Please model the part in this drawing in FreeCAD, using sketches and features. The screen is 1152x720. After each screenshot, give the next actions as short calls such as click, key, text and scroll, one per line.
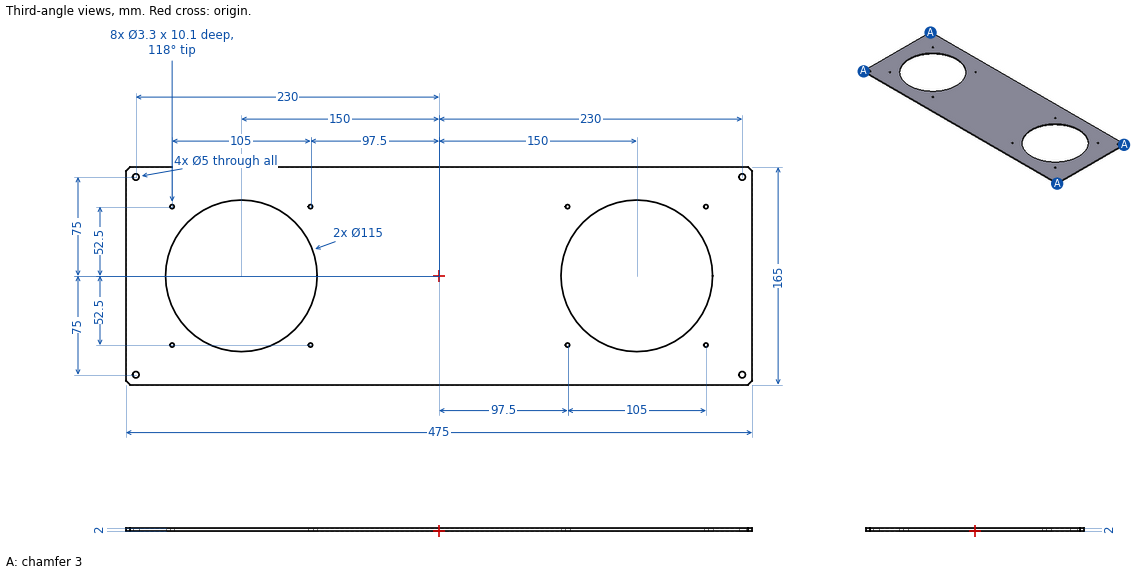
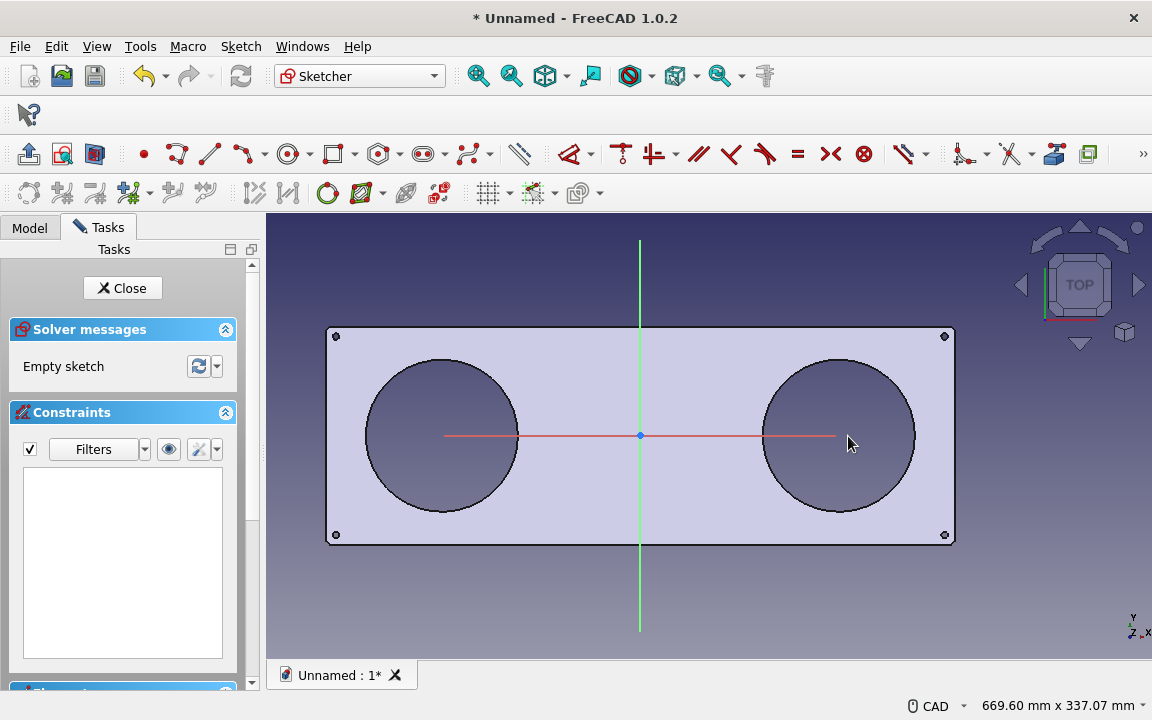
click(288, 154)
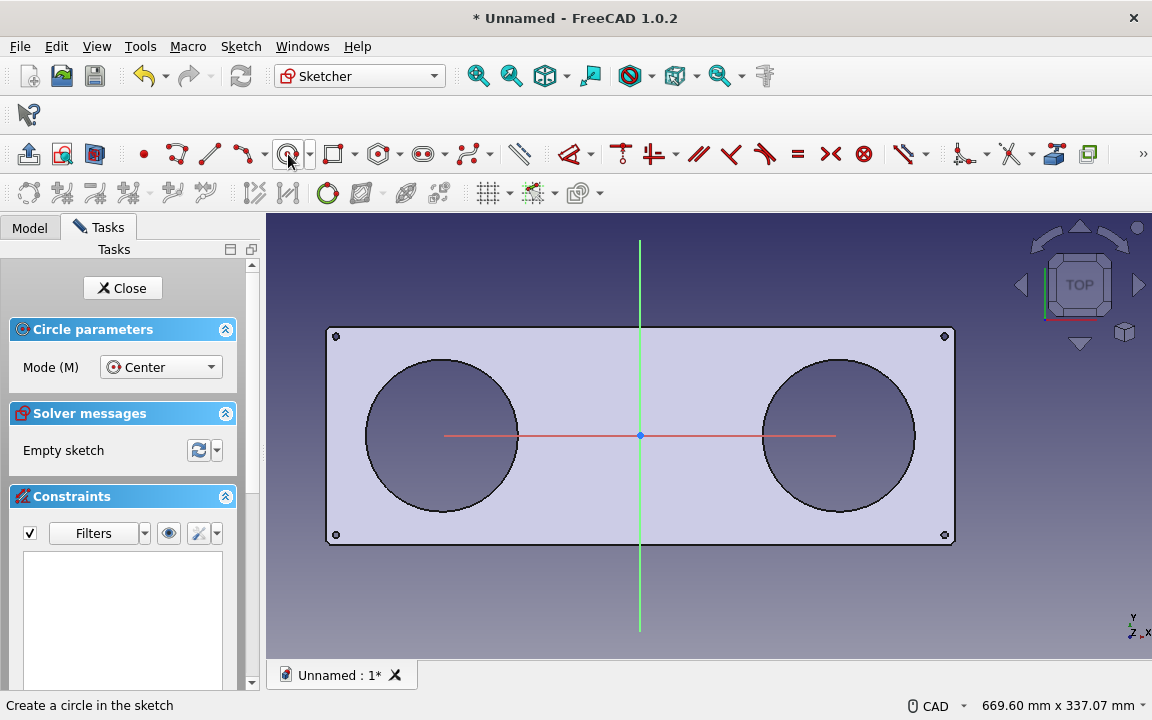
scroll(372, 366, up, 12)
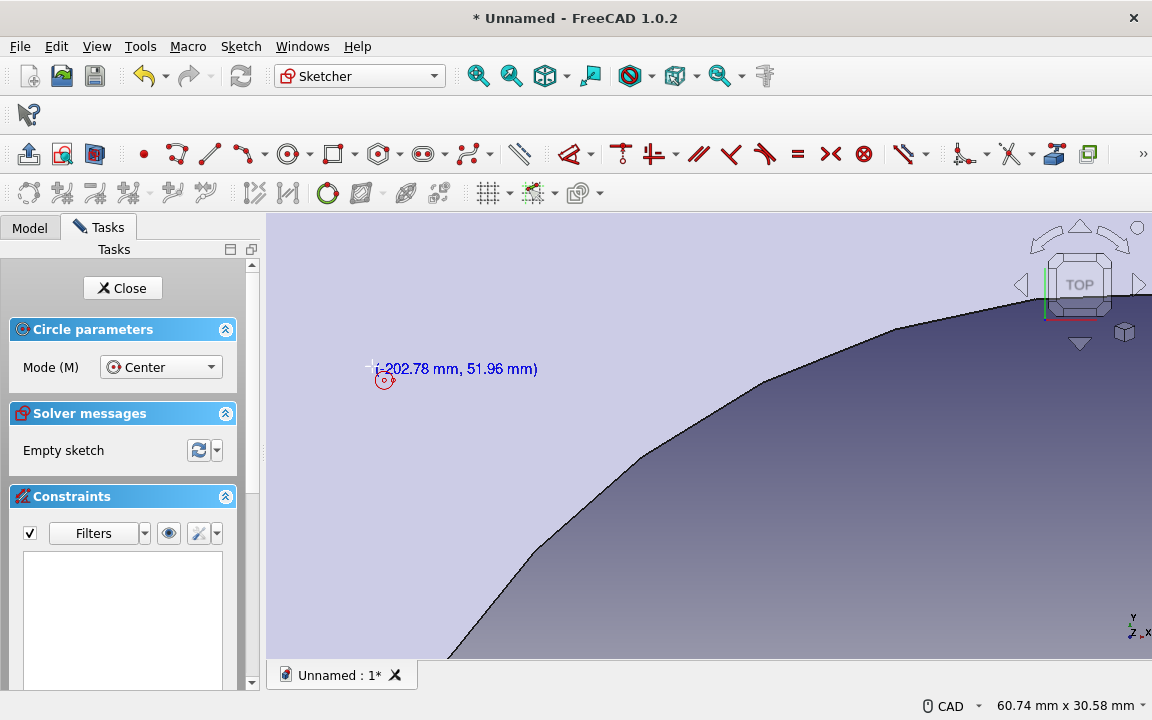
scroll(372, 367, down, 12)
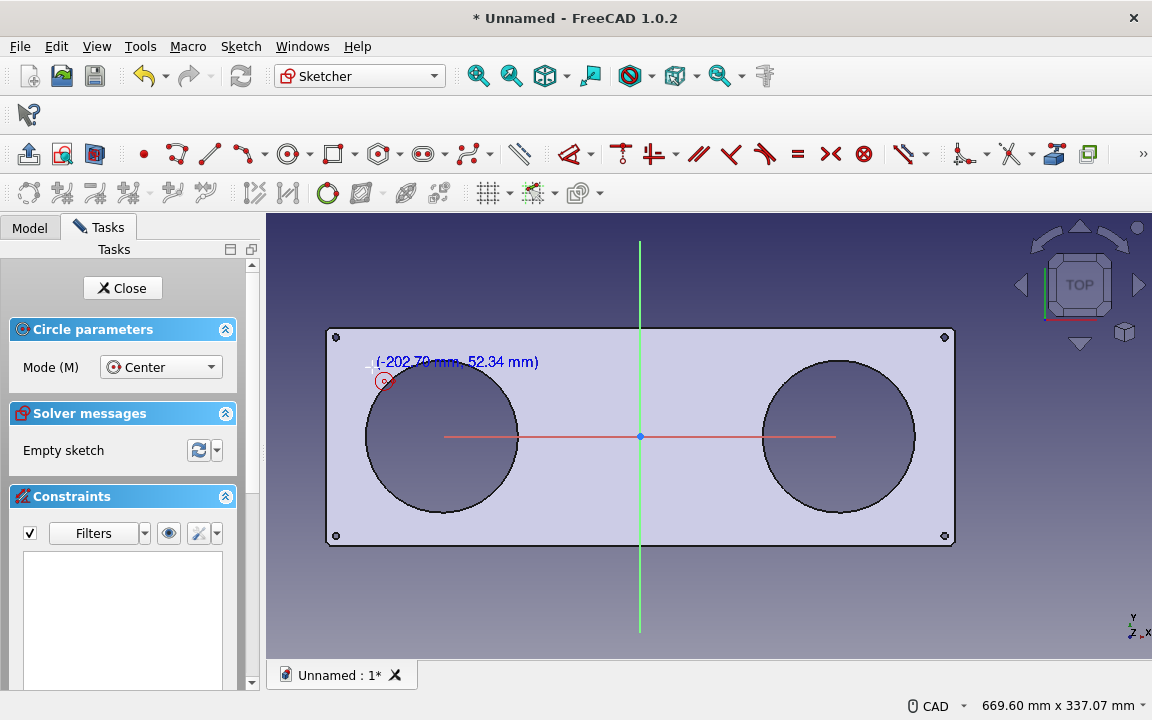
click(372, 367)
move(374, 366)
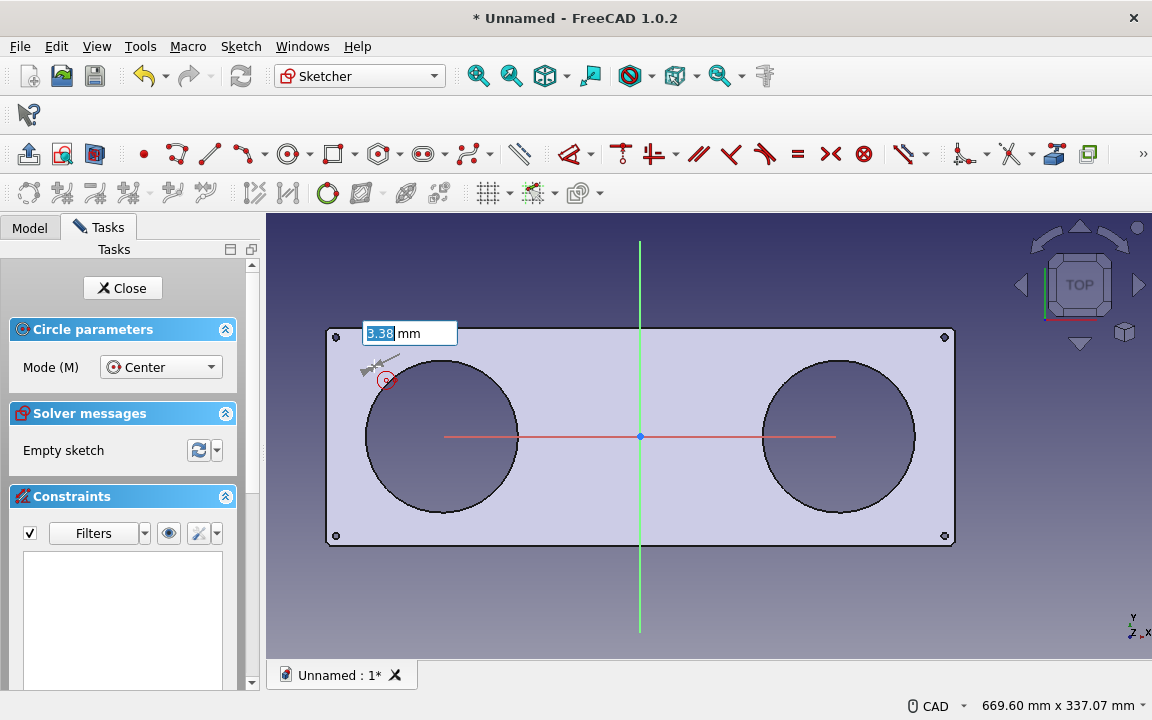
text(3.3)
key(Return)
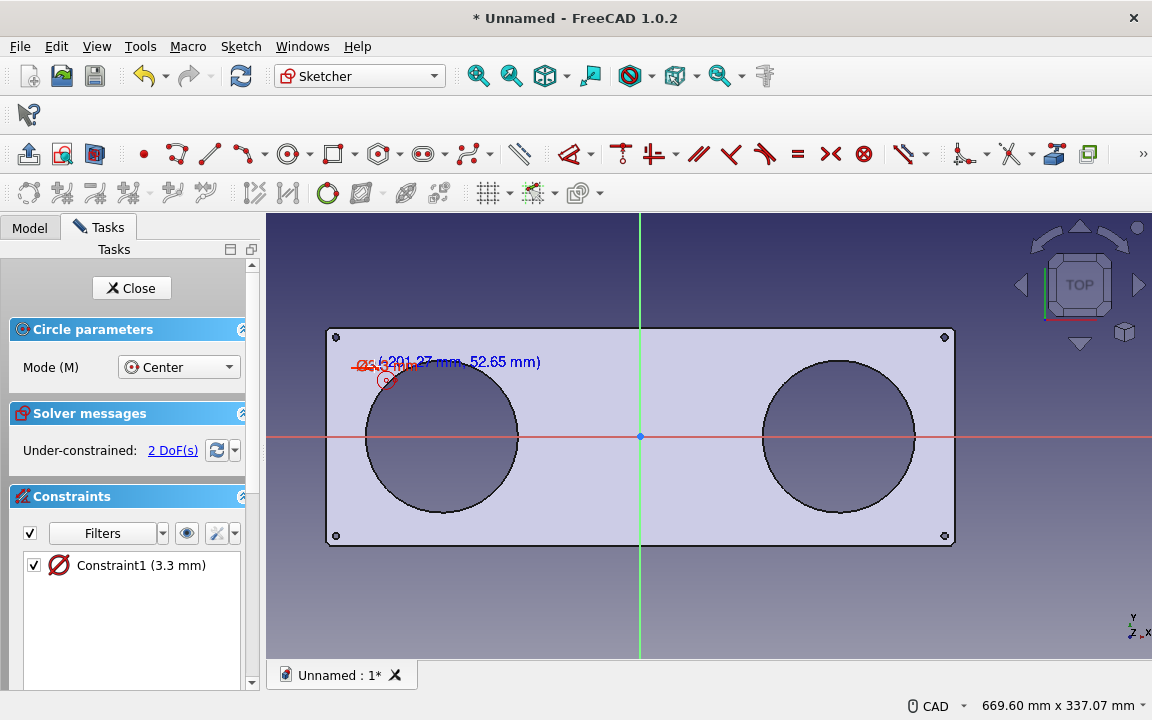
scroll(511, 367, up, 12)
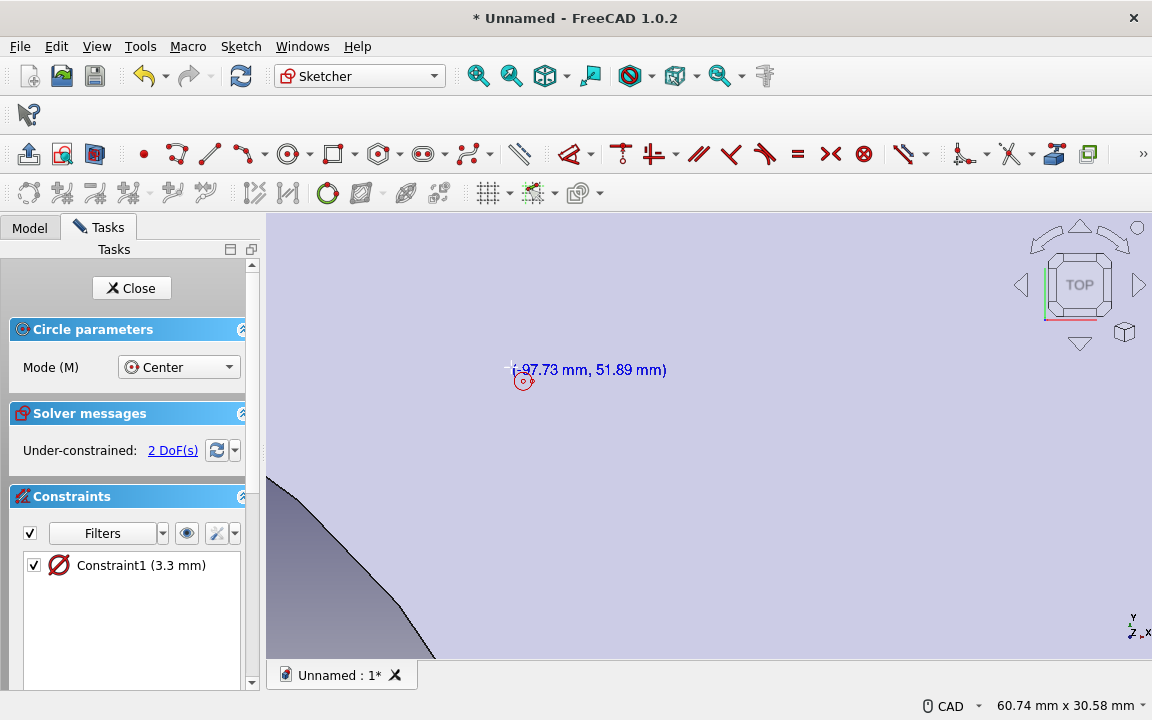
scroll(511, 367, down, 12)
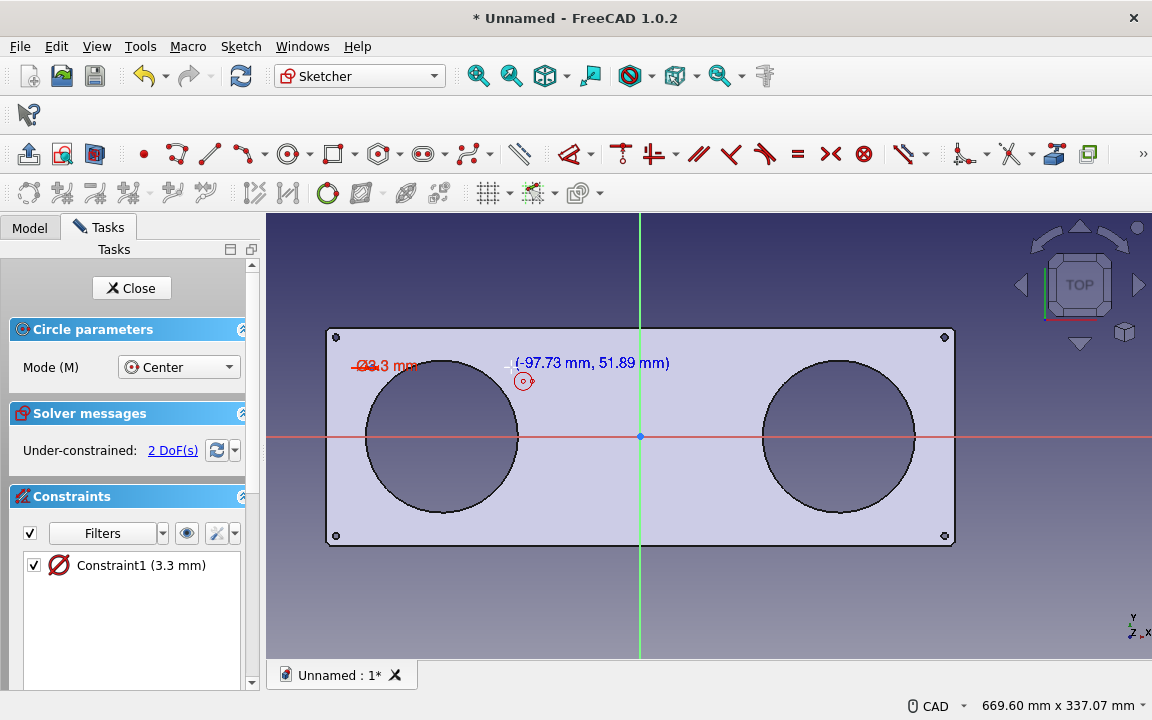
click(511, 367)
move(513, 366)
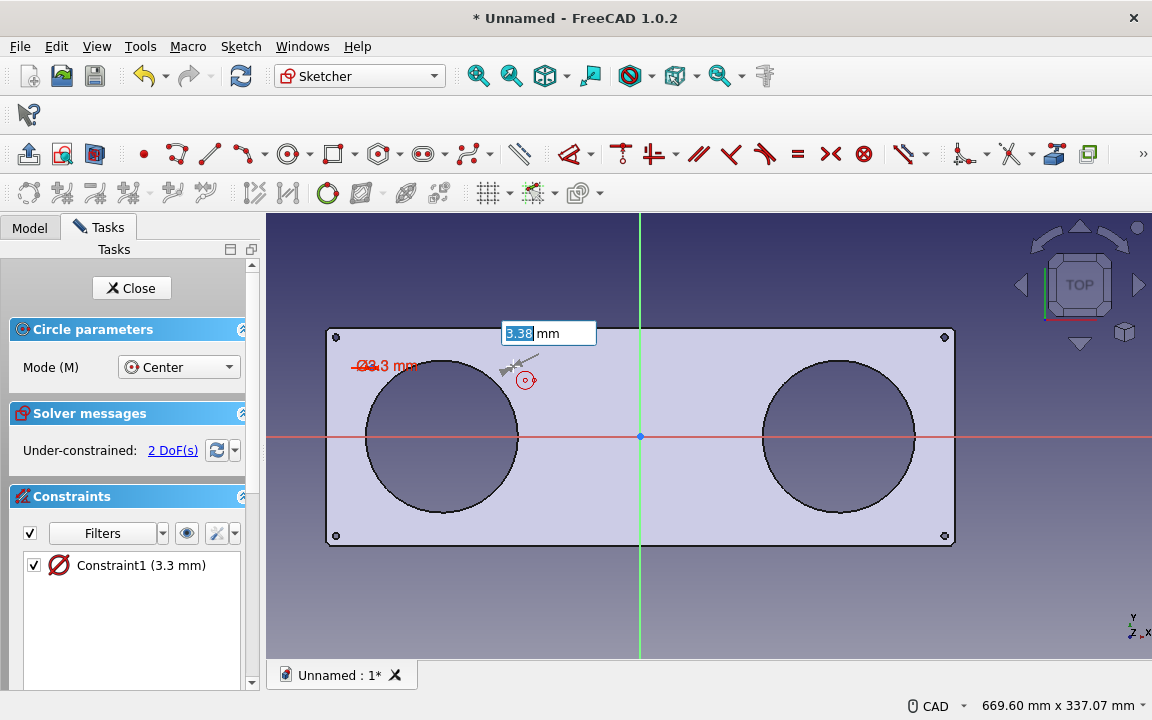
text(3.3)
key(Return)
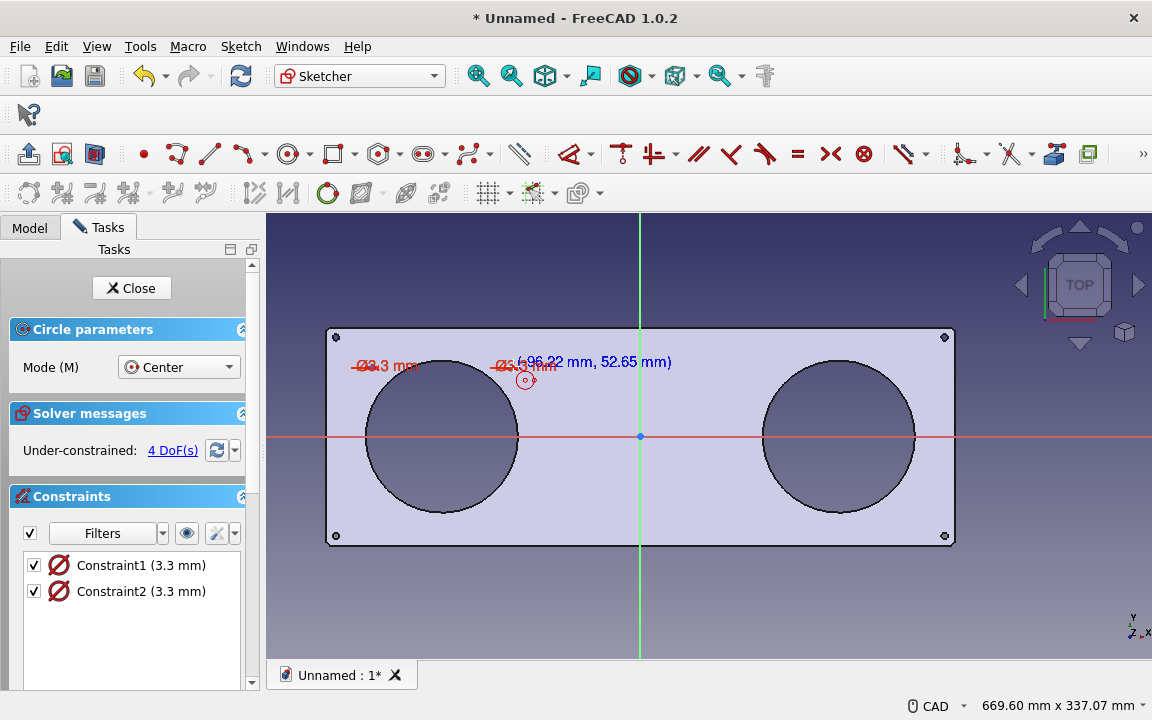
scroll(511, 506, up, 12)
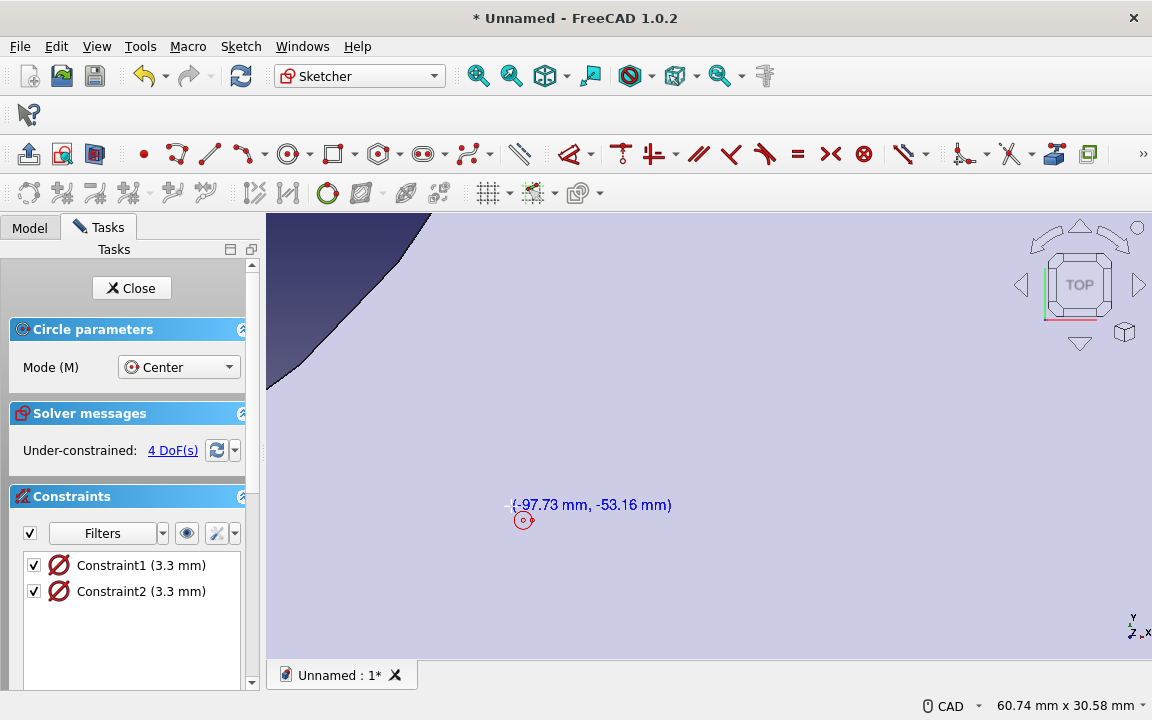
scroll(511, 506, down, 12)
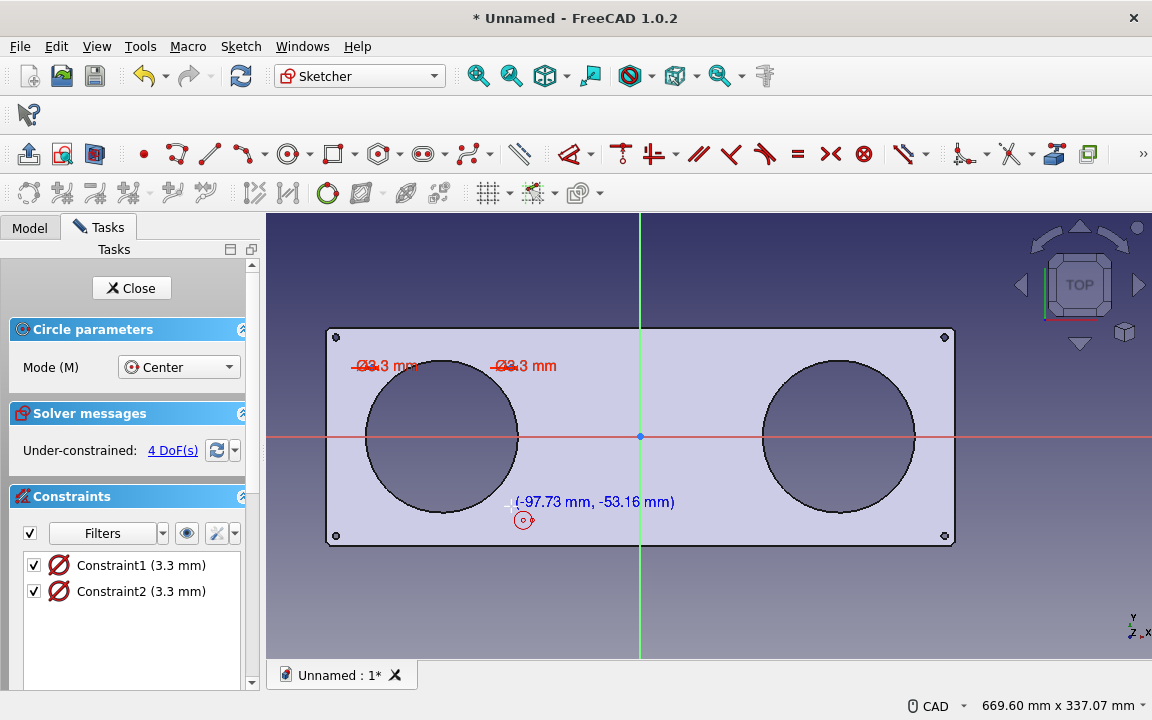
click(511, 506)
move(513, 505)